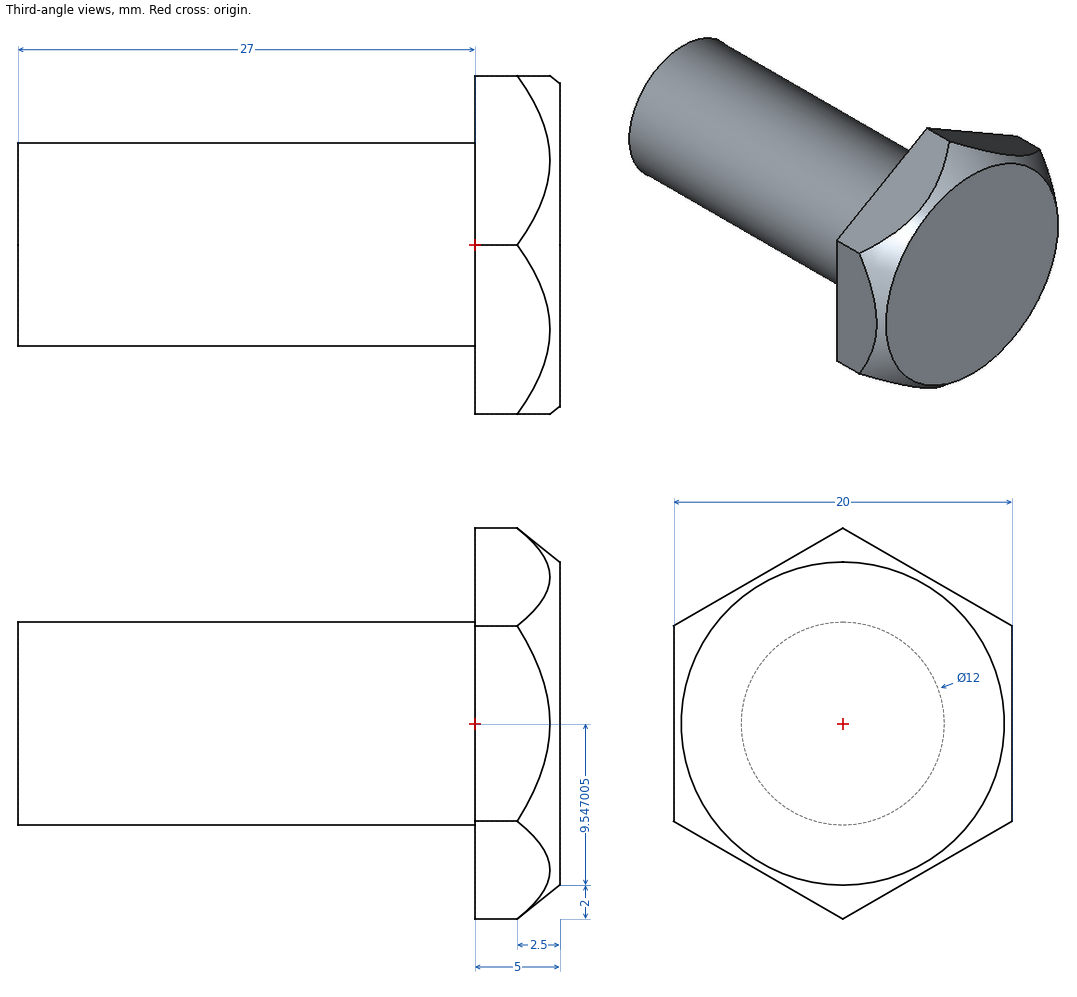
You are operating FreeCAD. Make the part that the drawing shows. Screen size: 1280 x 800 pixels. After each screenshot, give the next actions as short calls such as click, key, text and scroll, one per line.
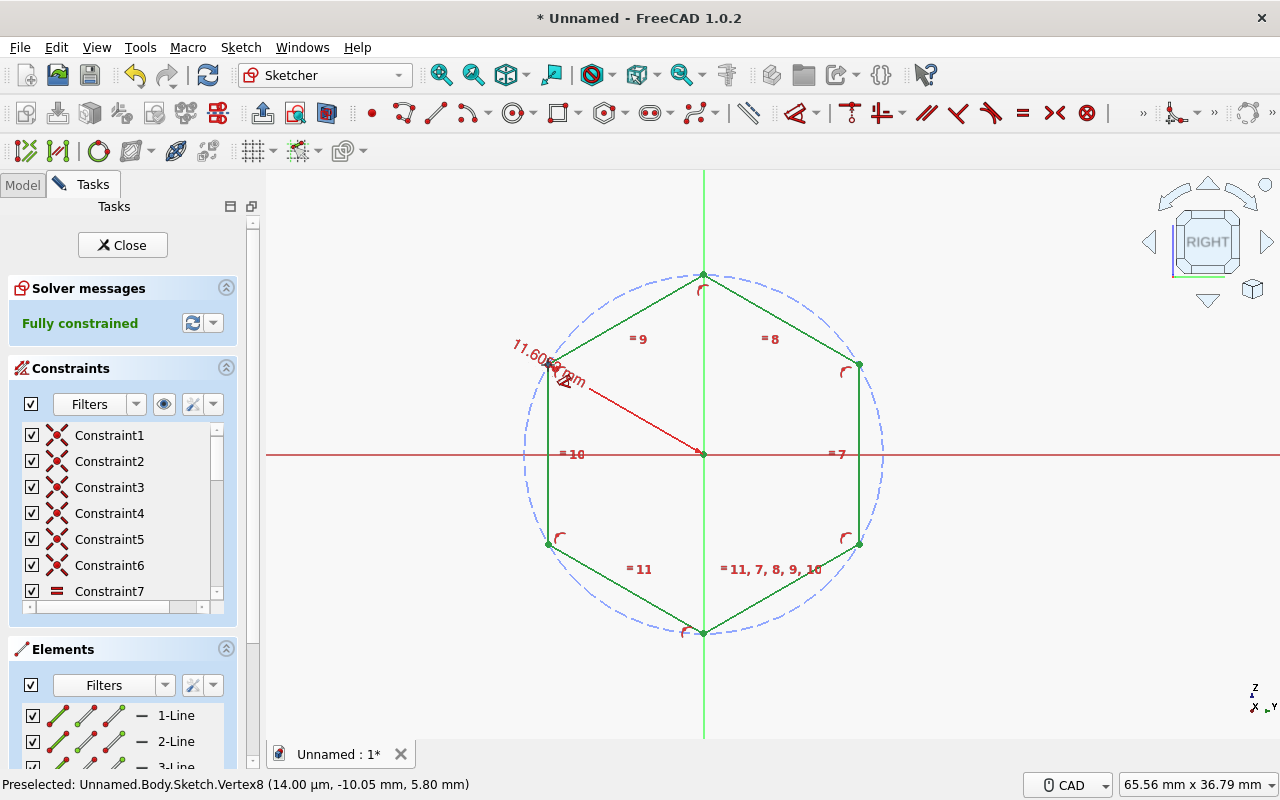
click(859, 544)
click(595, 626)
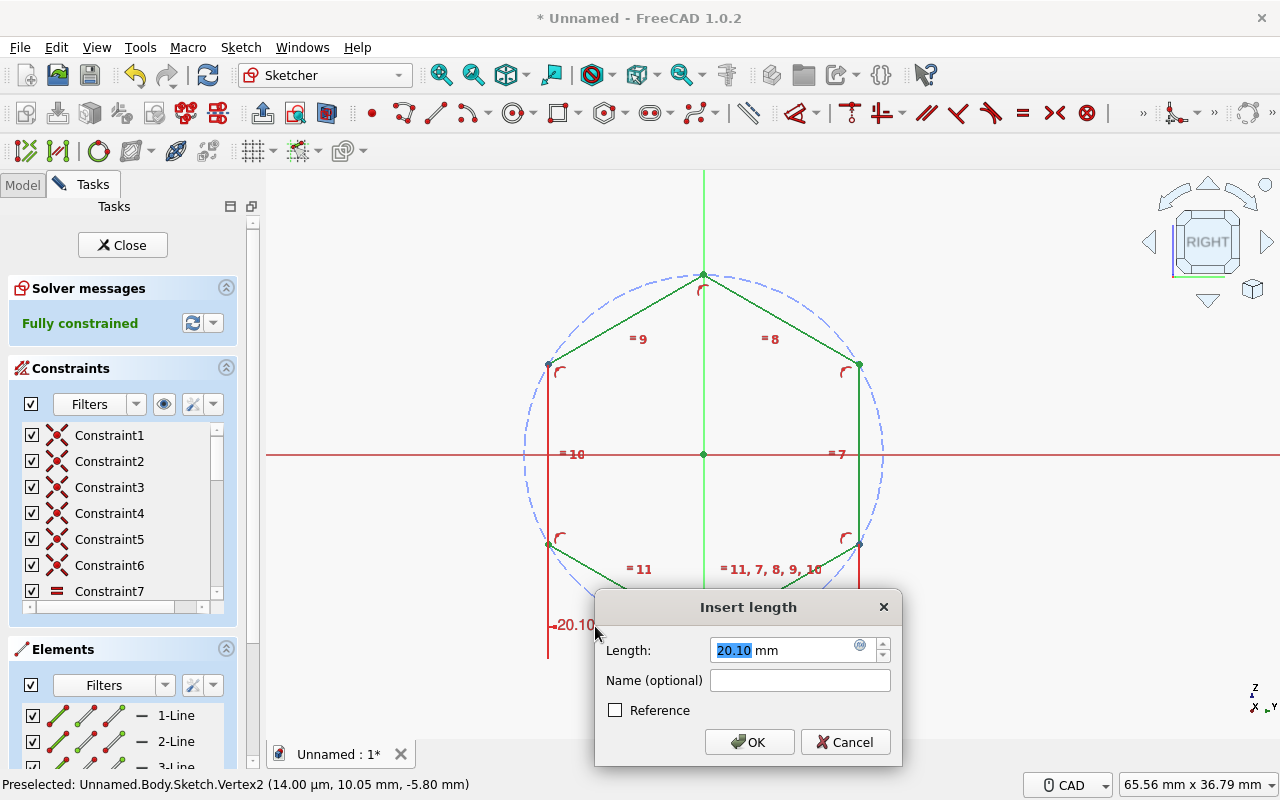
text(20)
key(Return)
key(Escape)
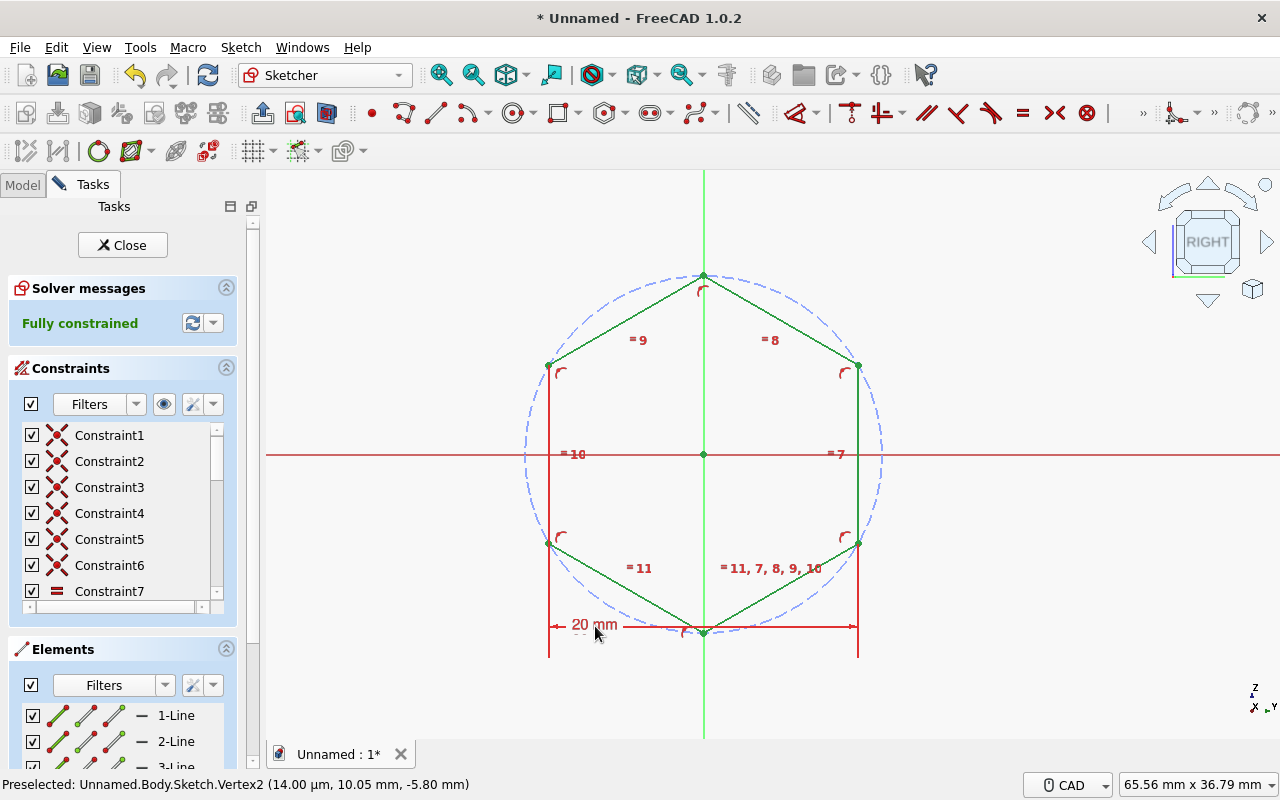
click(123, 245)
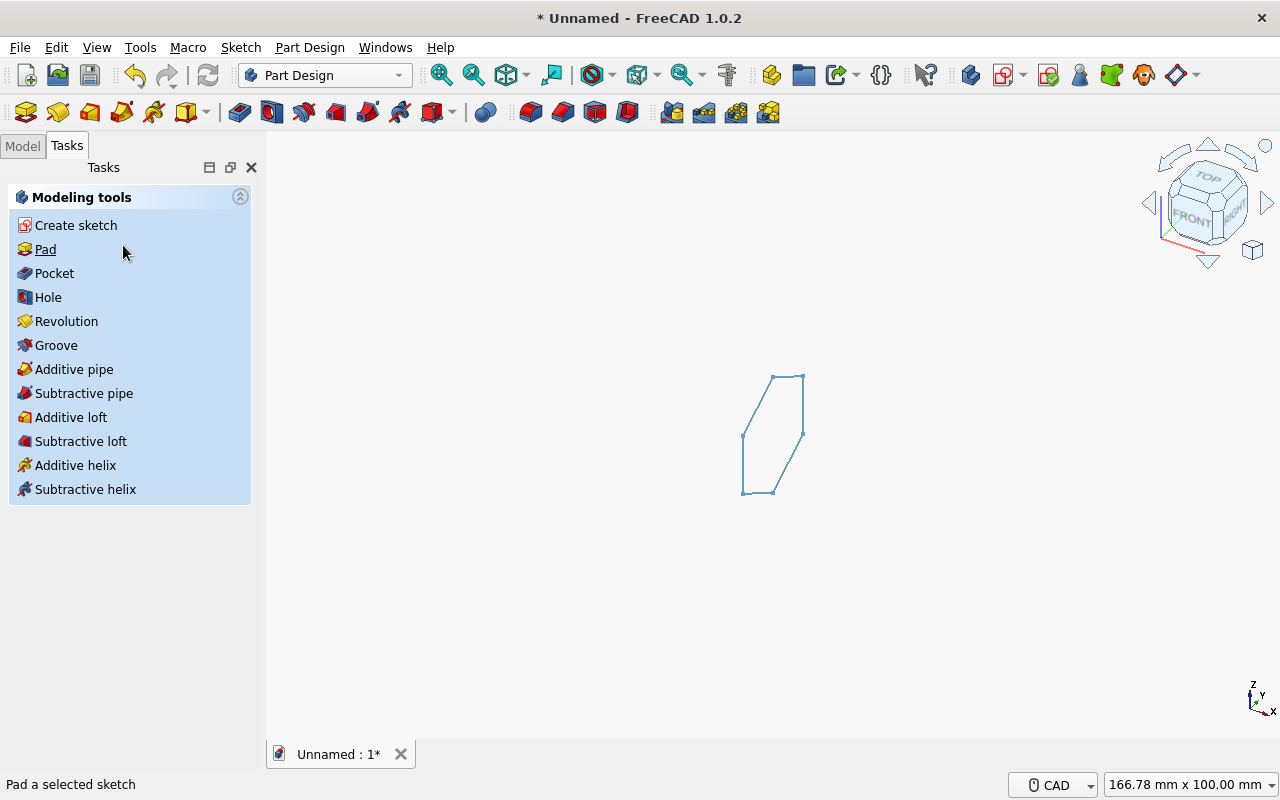
click(26, 112)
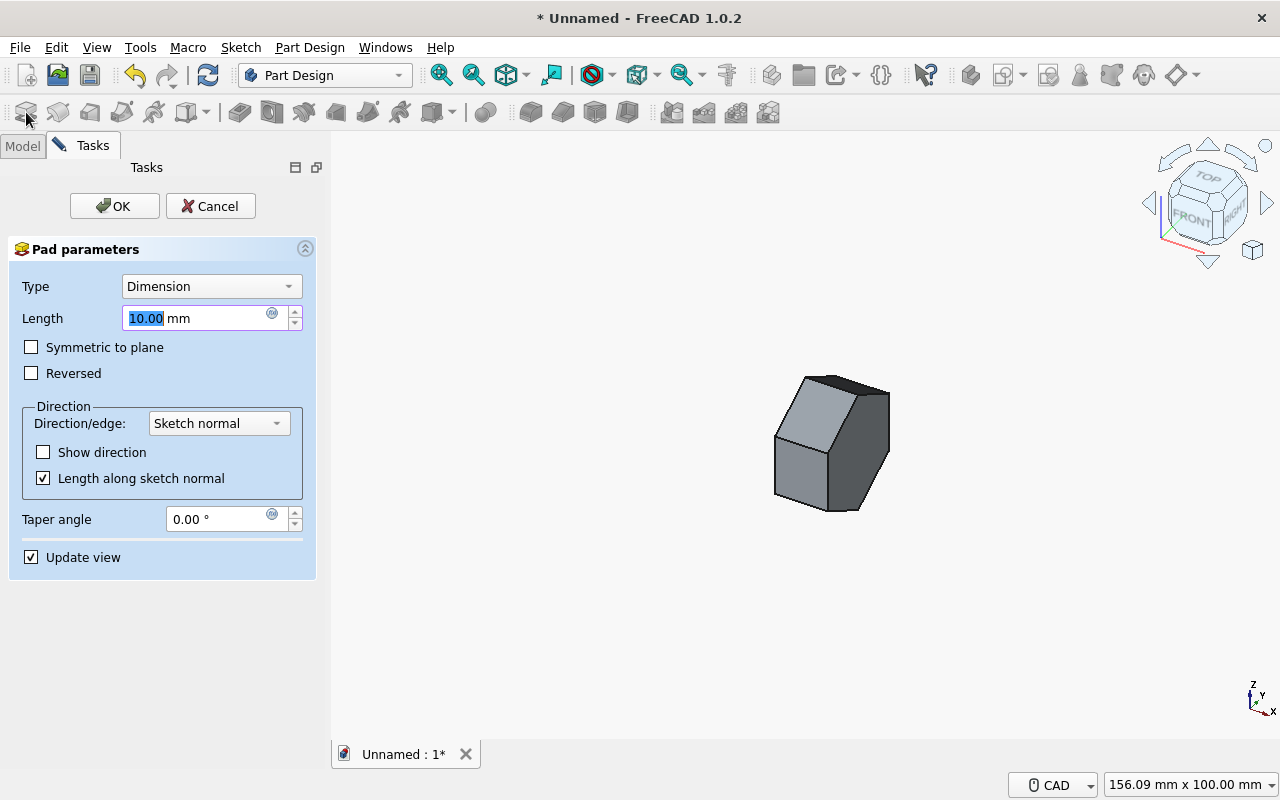
text(5)
key(Tab)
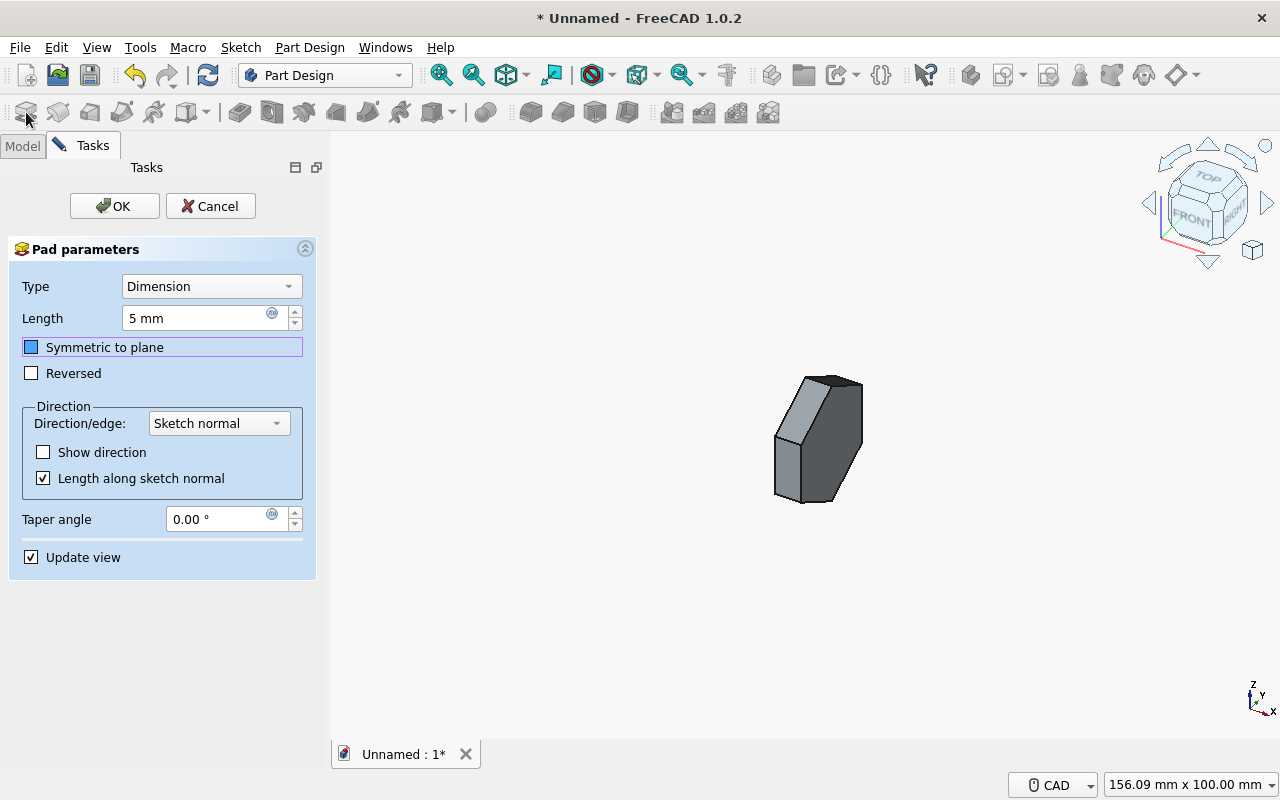
click(115, 206)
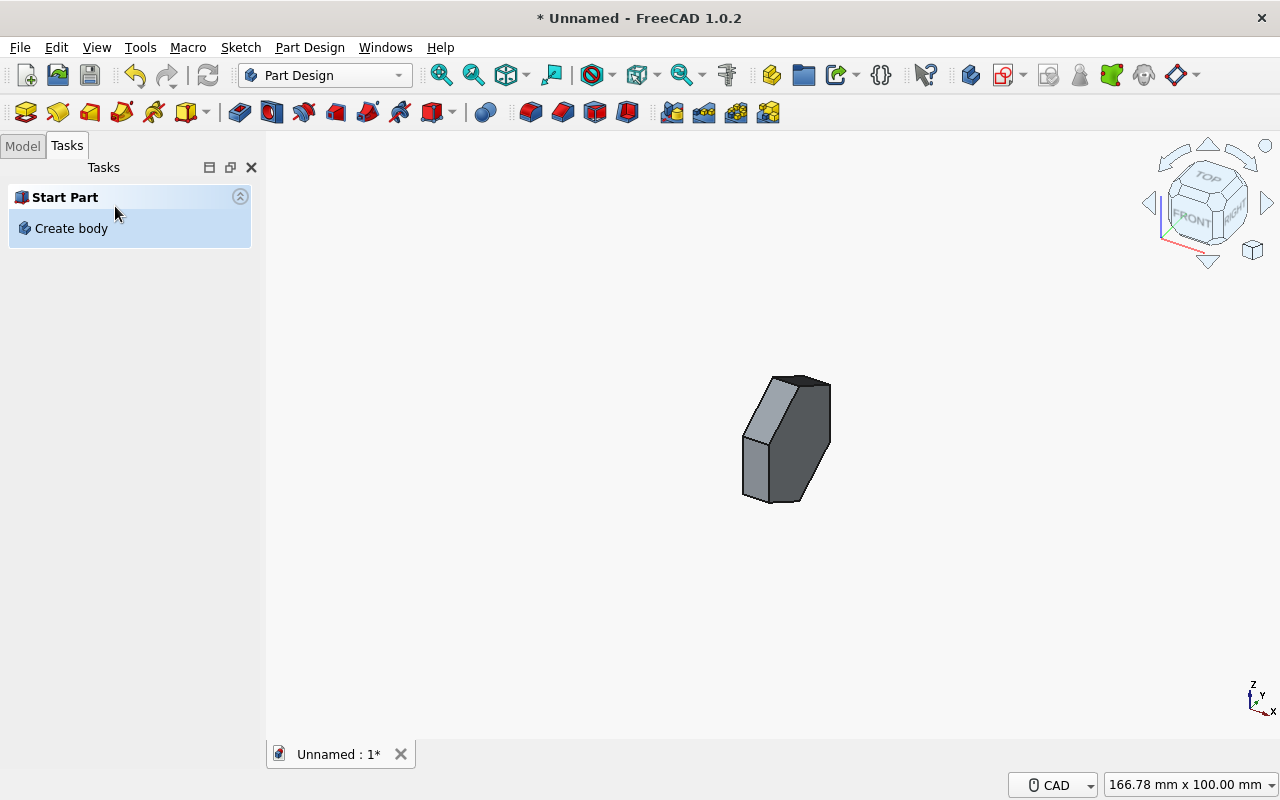
click(442, 76)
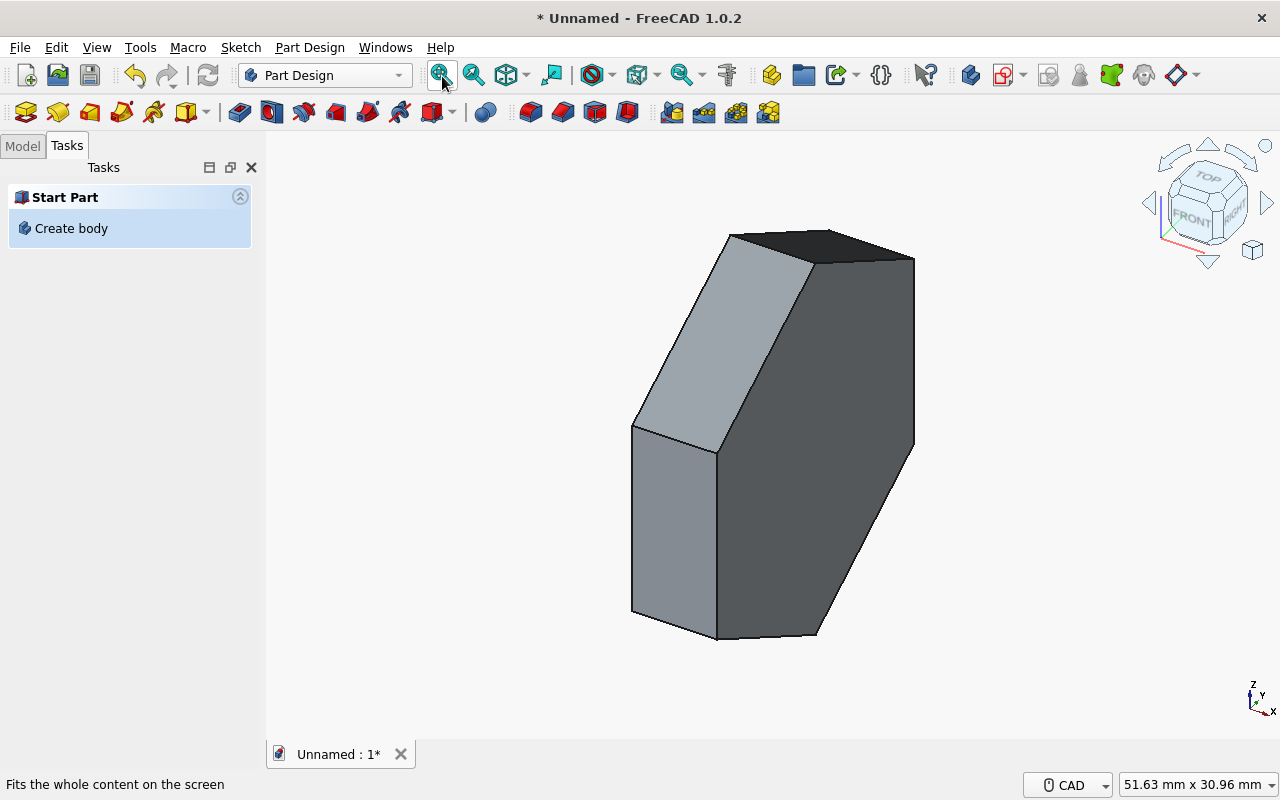
key(6)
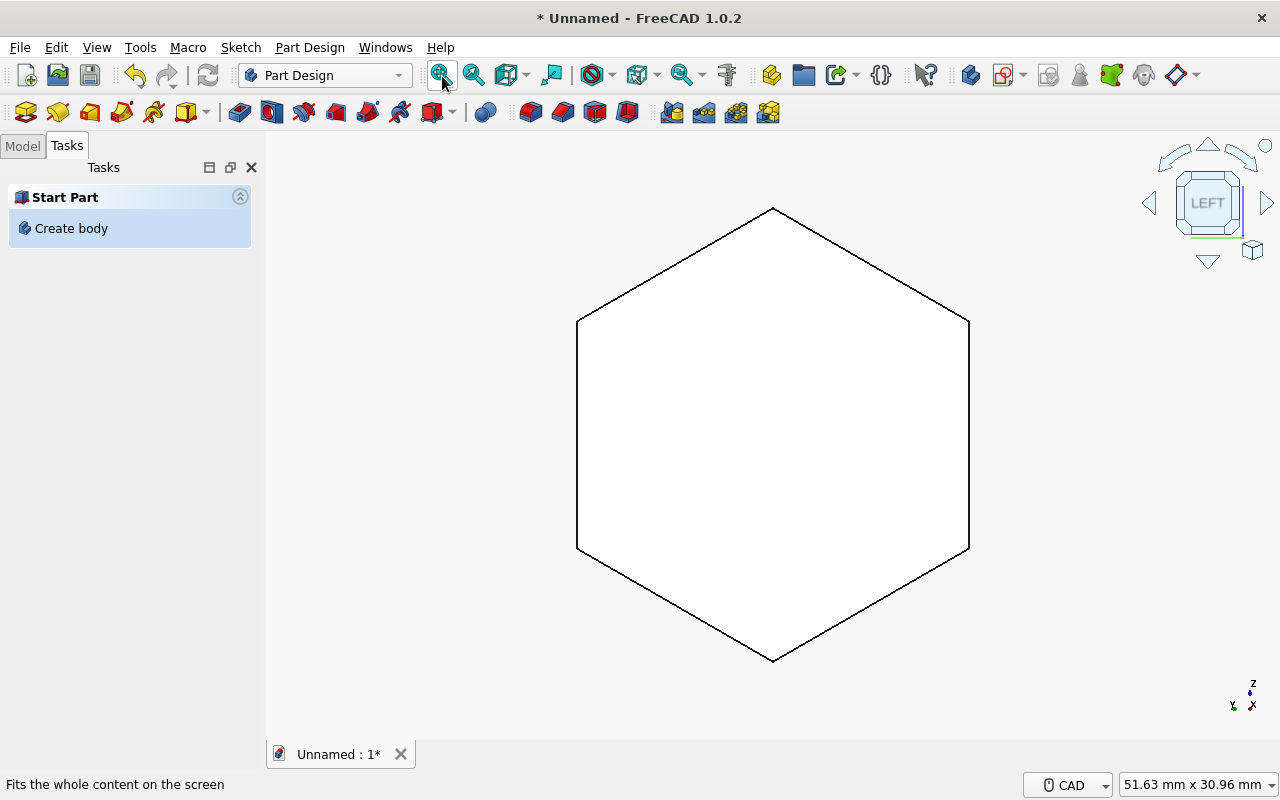
click(773, 434)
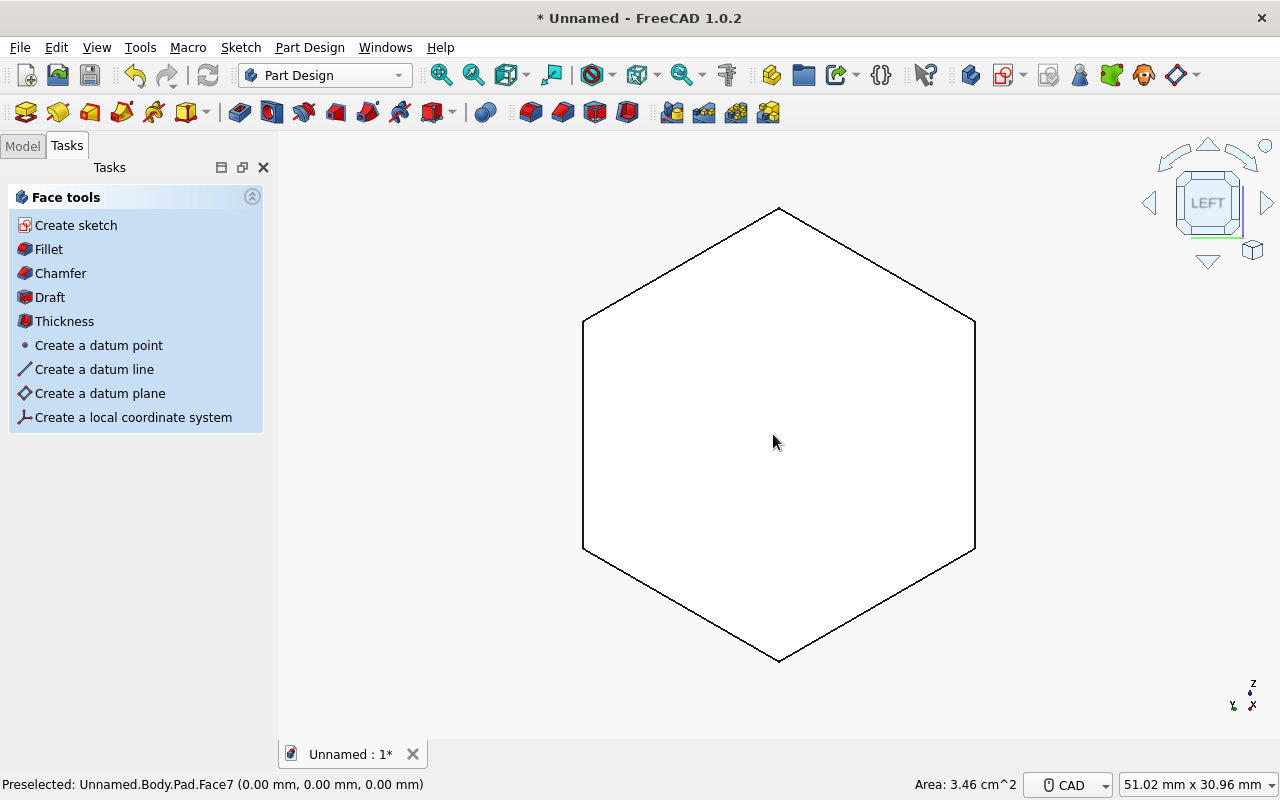
click(1004, 76)